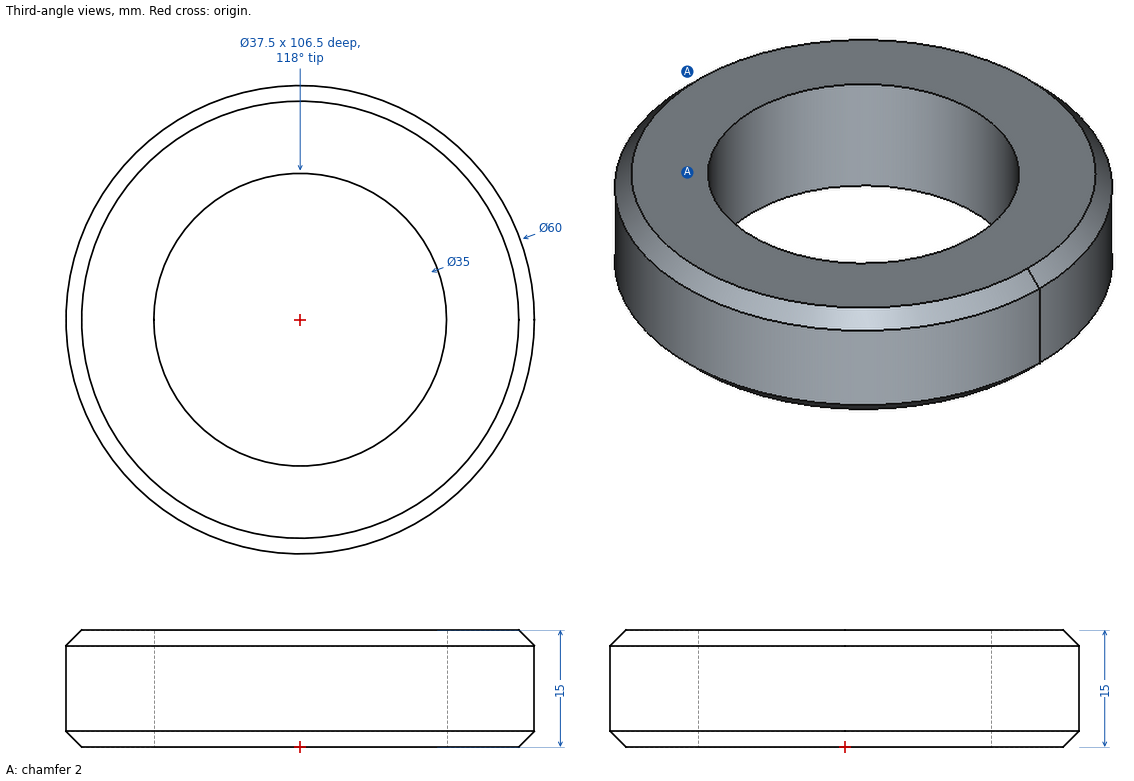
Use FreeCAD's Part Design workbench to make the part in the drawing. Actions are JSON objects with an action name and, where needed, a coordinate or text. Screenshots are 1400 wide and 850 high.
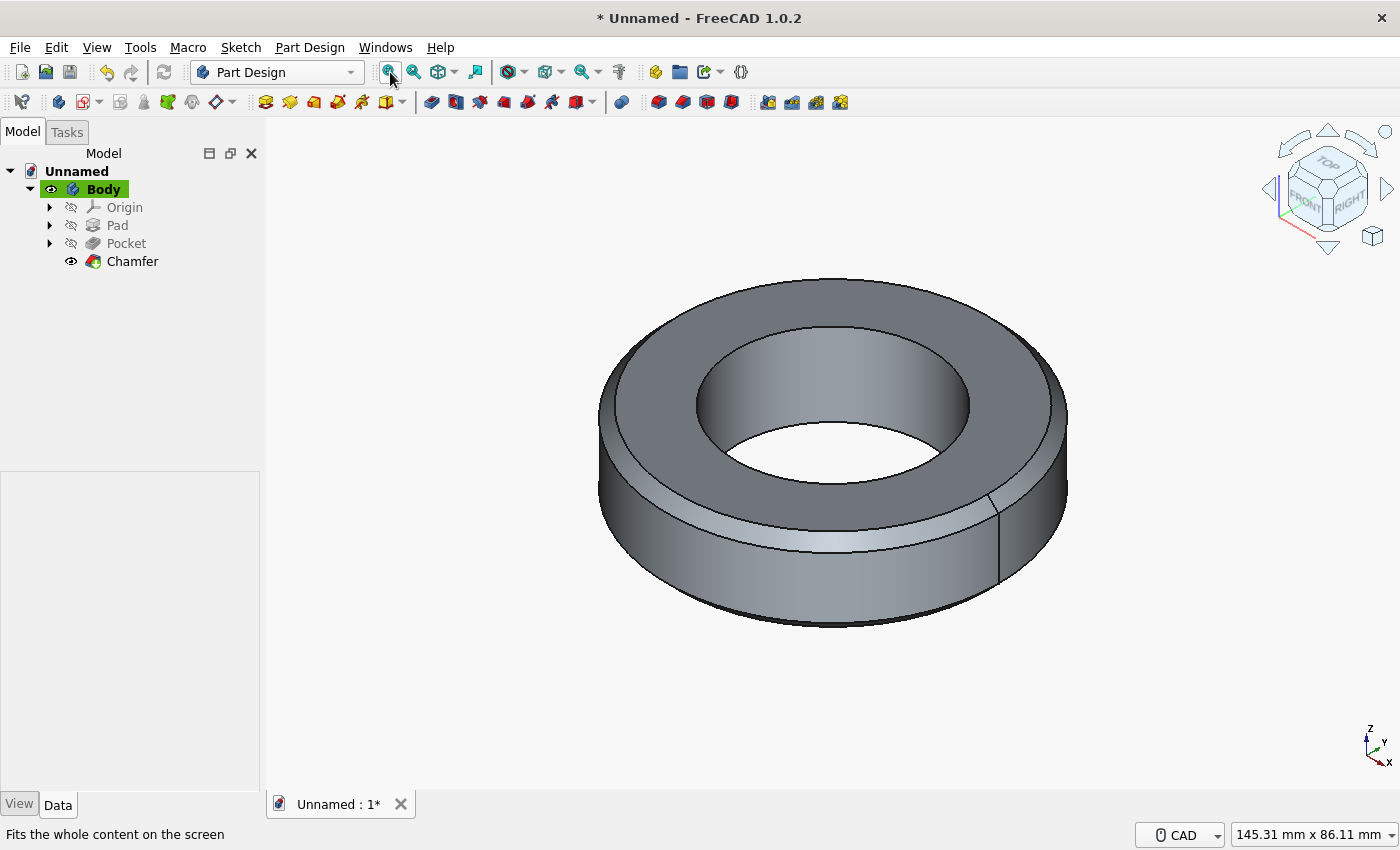
{"action": "left_click", "coordinate": [833, 302]}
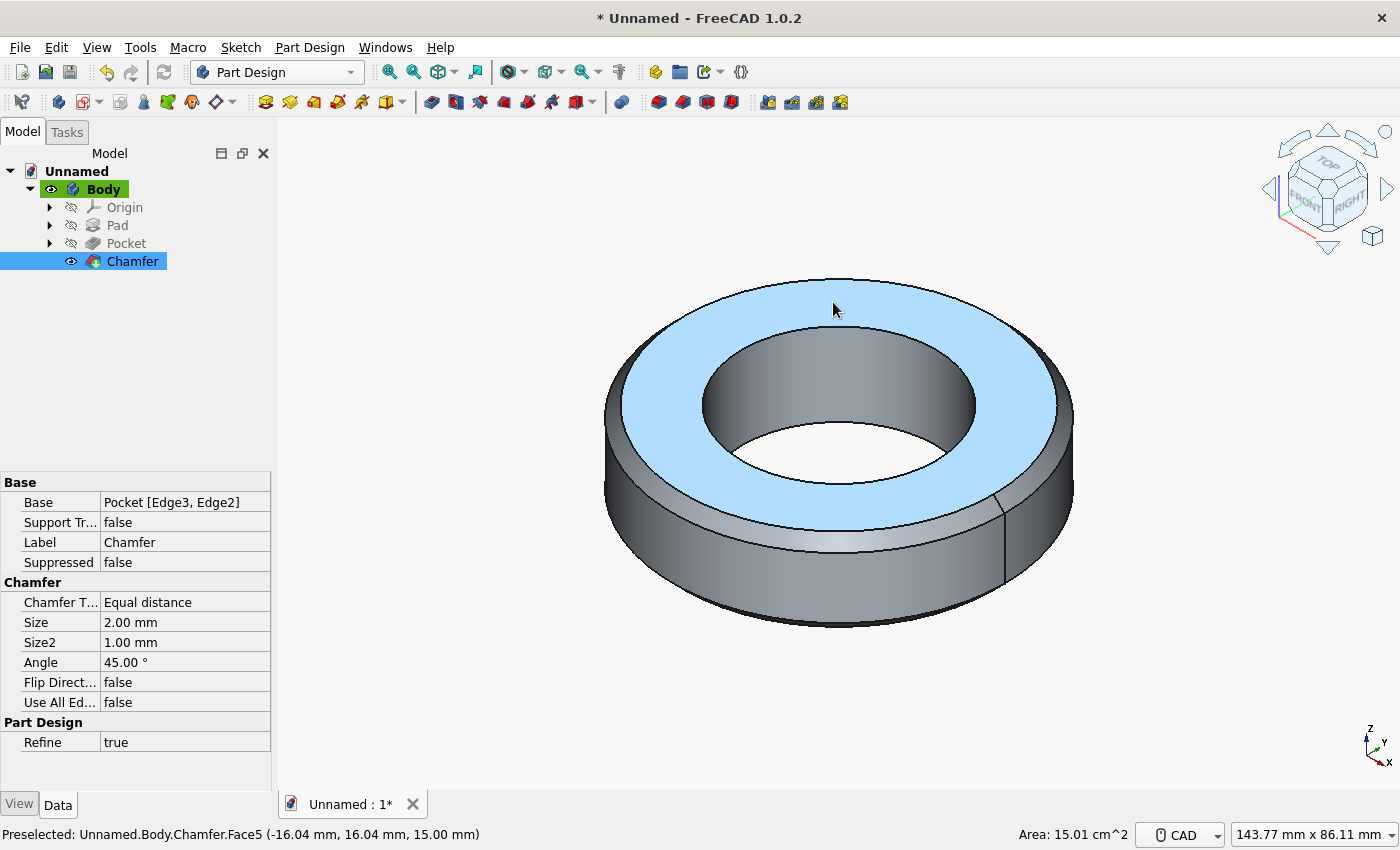
{"action": "left_click", "coordinate": [84, 102]}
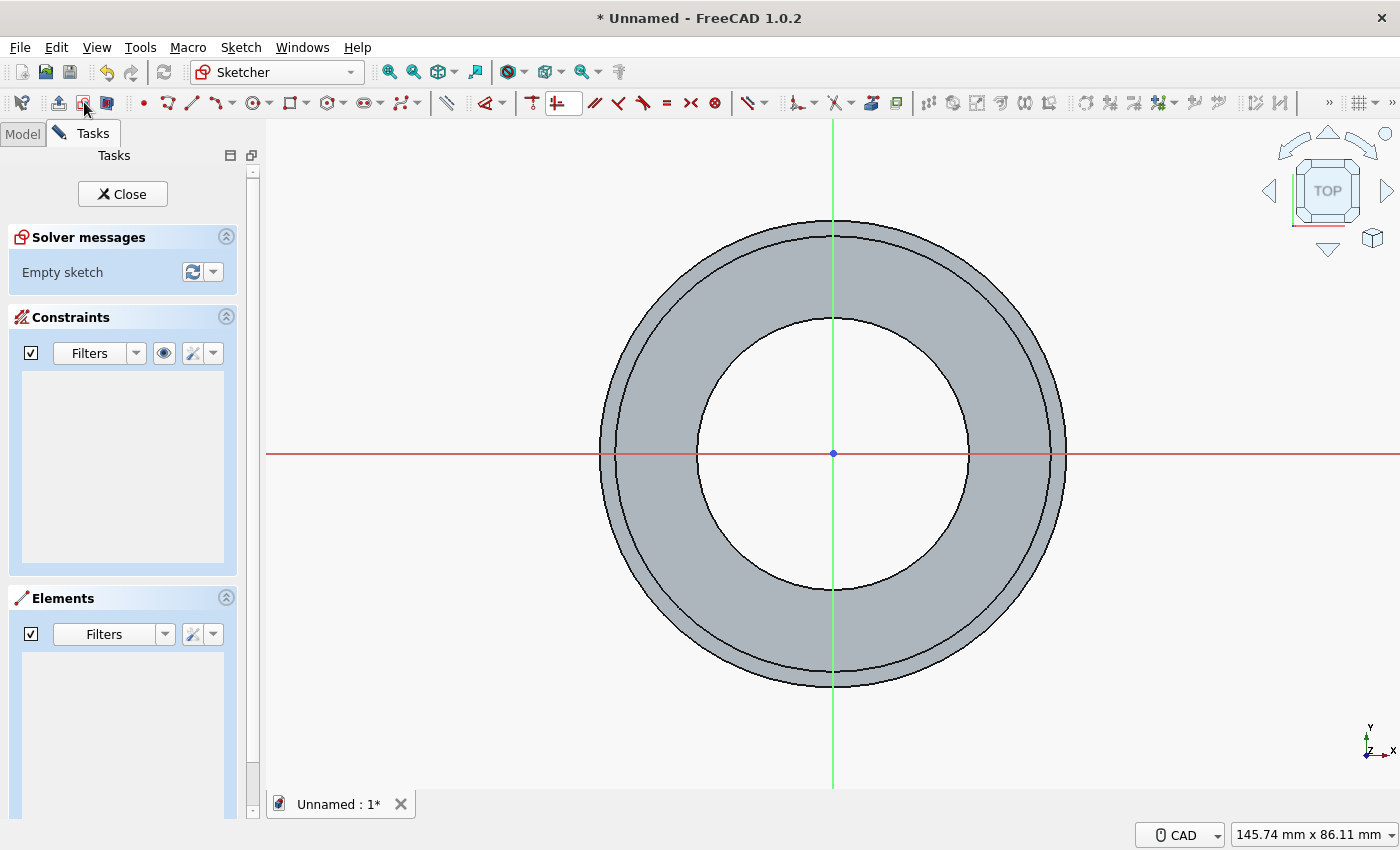
{"action": "scroll", "coordinate": [972, 454], "scroll_direction": "up", "scroll_amount": 2}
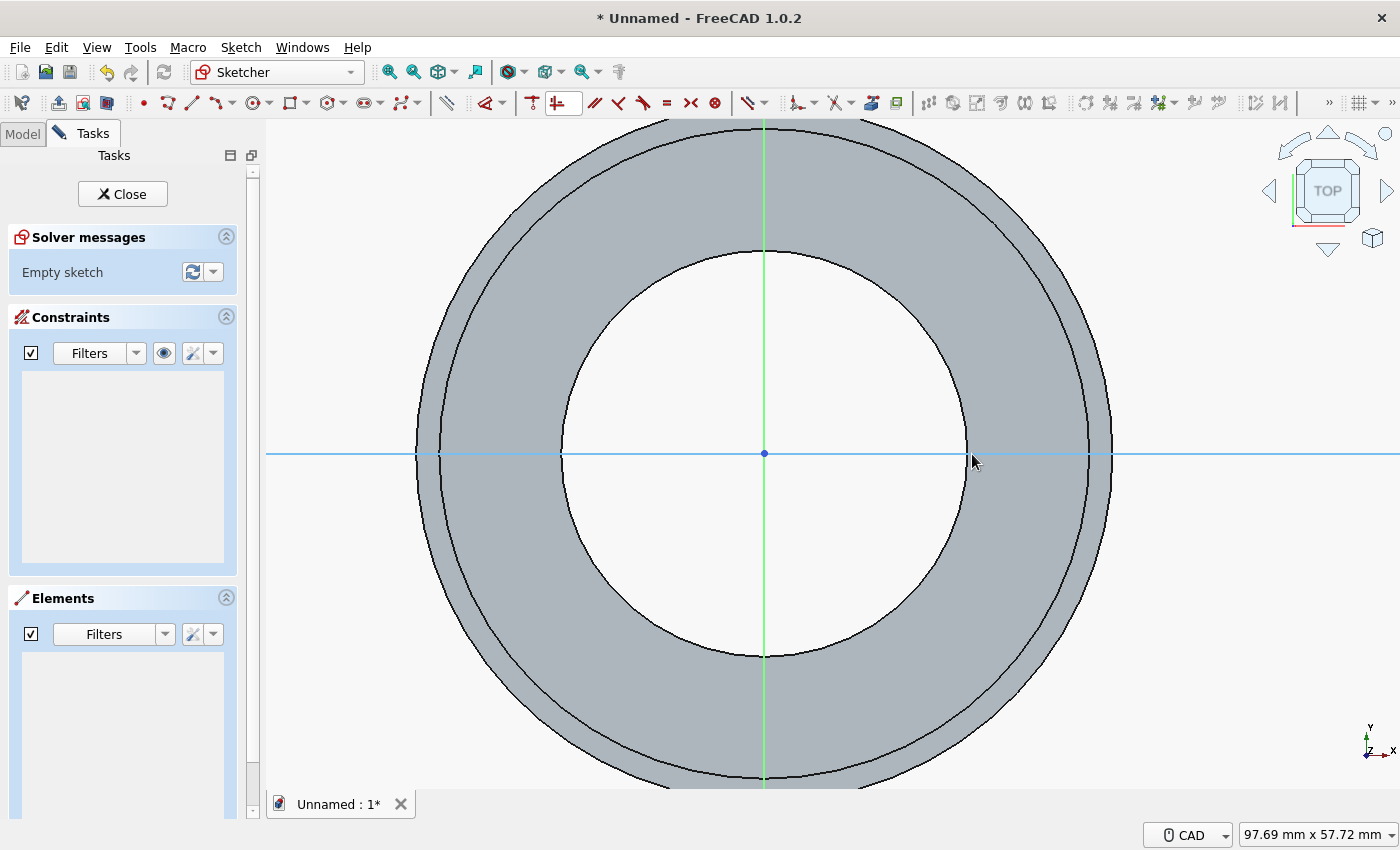
{"action": "left_click", "coordinate": [254, 104]}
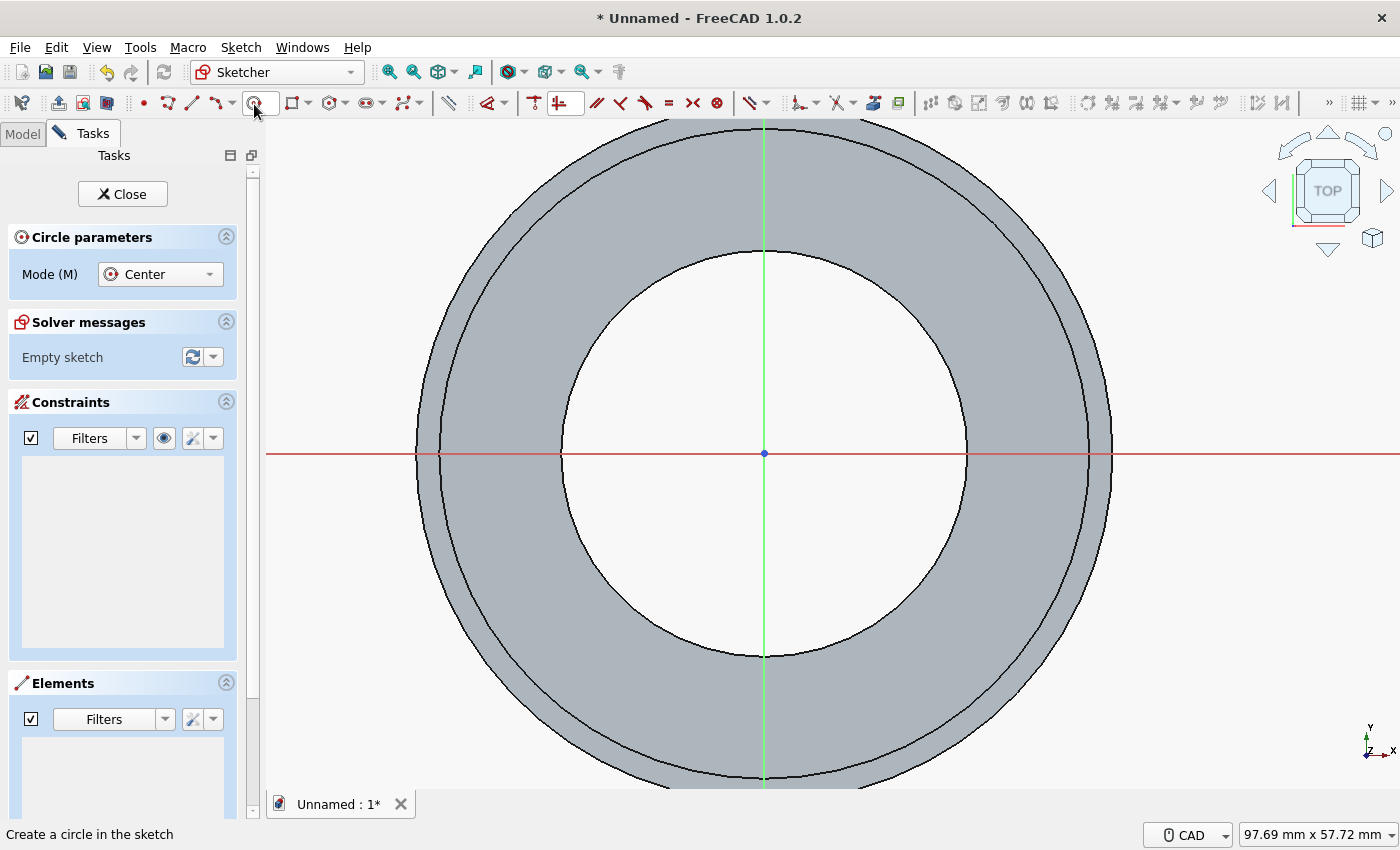
{"action": "left_click", "coordinate": [764, 454]}
{"action": "mouse_move", "coordinate": [918, 300]}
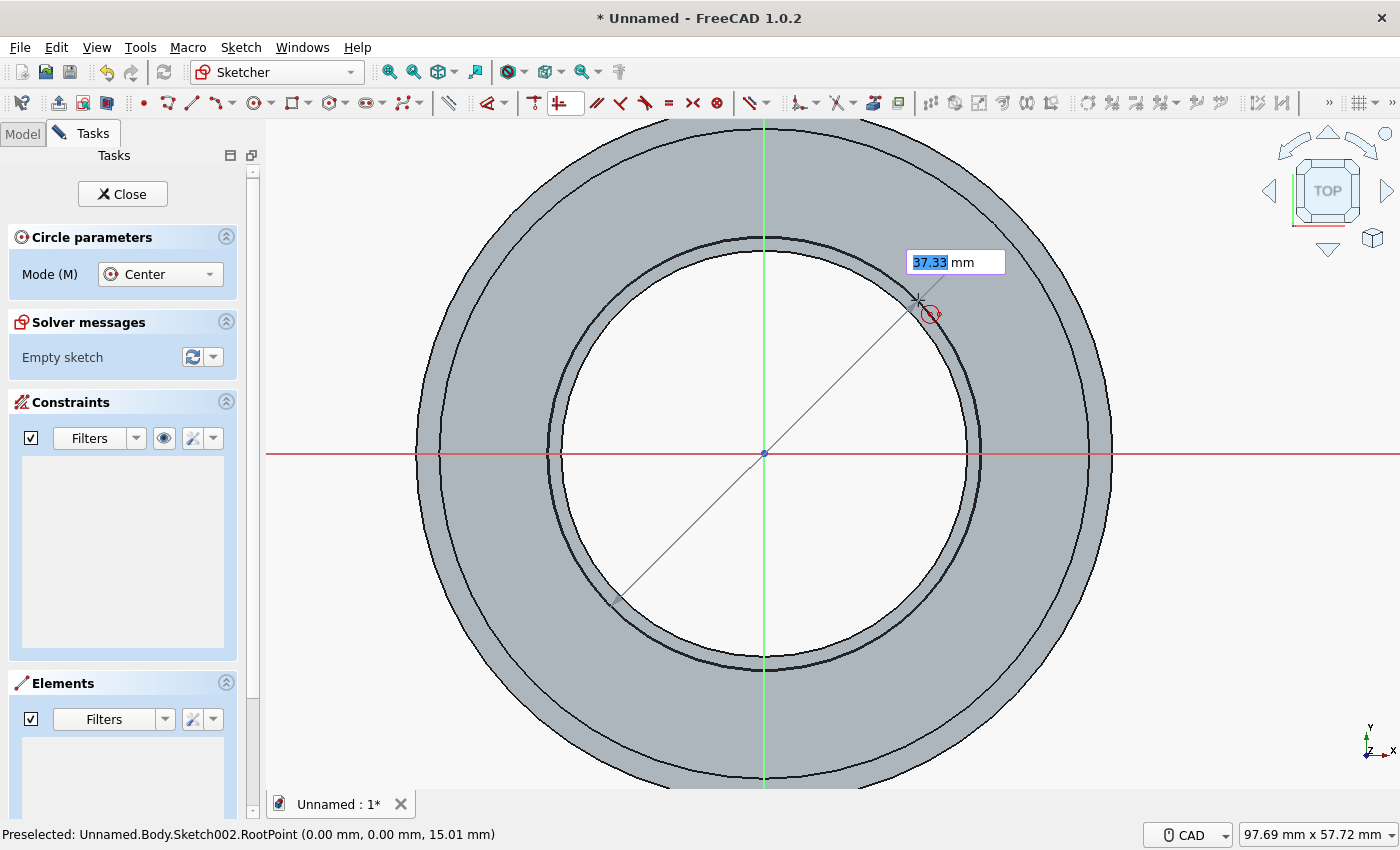
{"action": "type", "text": "37.5"}
{"action": "key", "text": "Return"}
{"action": "key", "text": "Escape"}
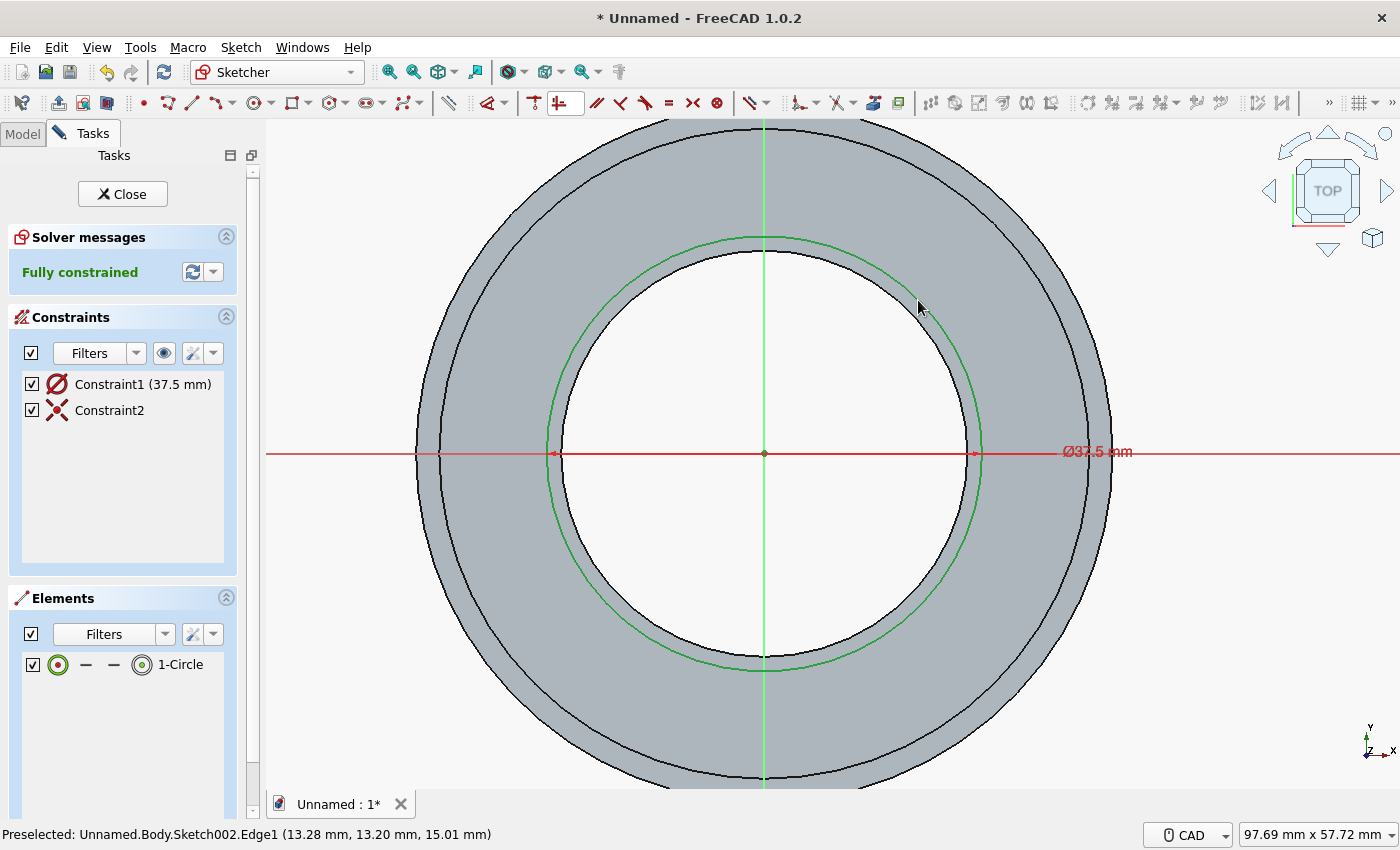
{"action": "left_click", "coordinate": [123, 194]}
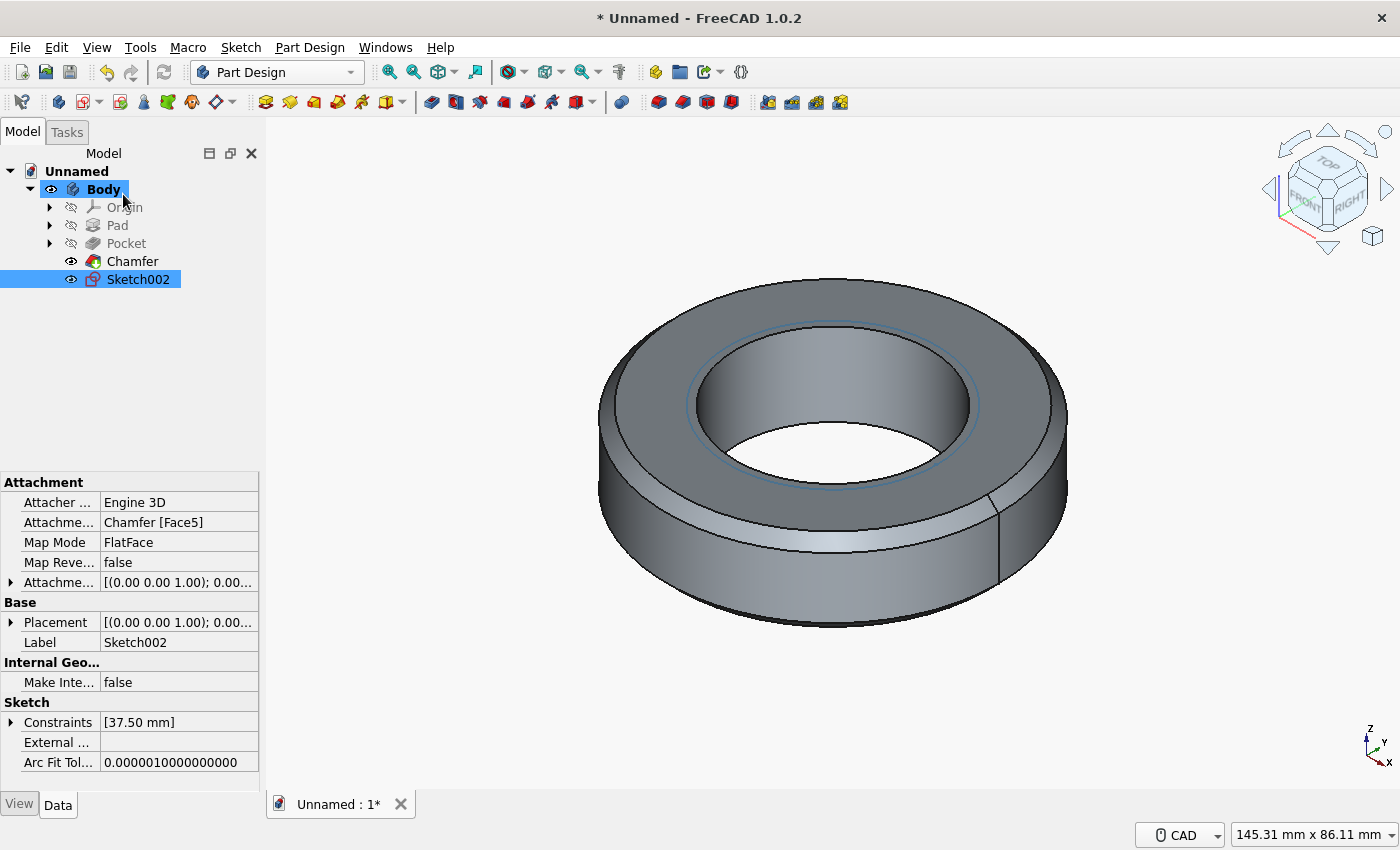
{"action": "left_click", "coordinate": [456, 102]}